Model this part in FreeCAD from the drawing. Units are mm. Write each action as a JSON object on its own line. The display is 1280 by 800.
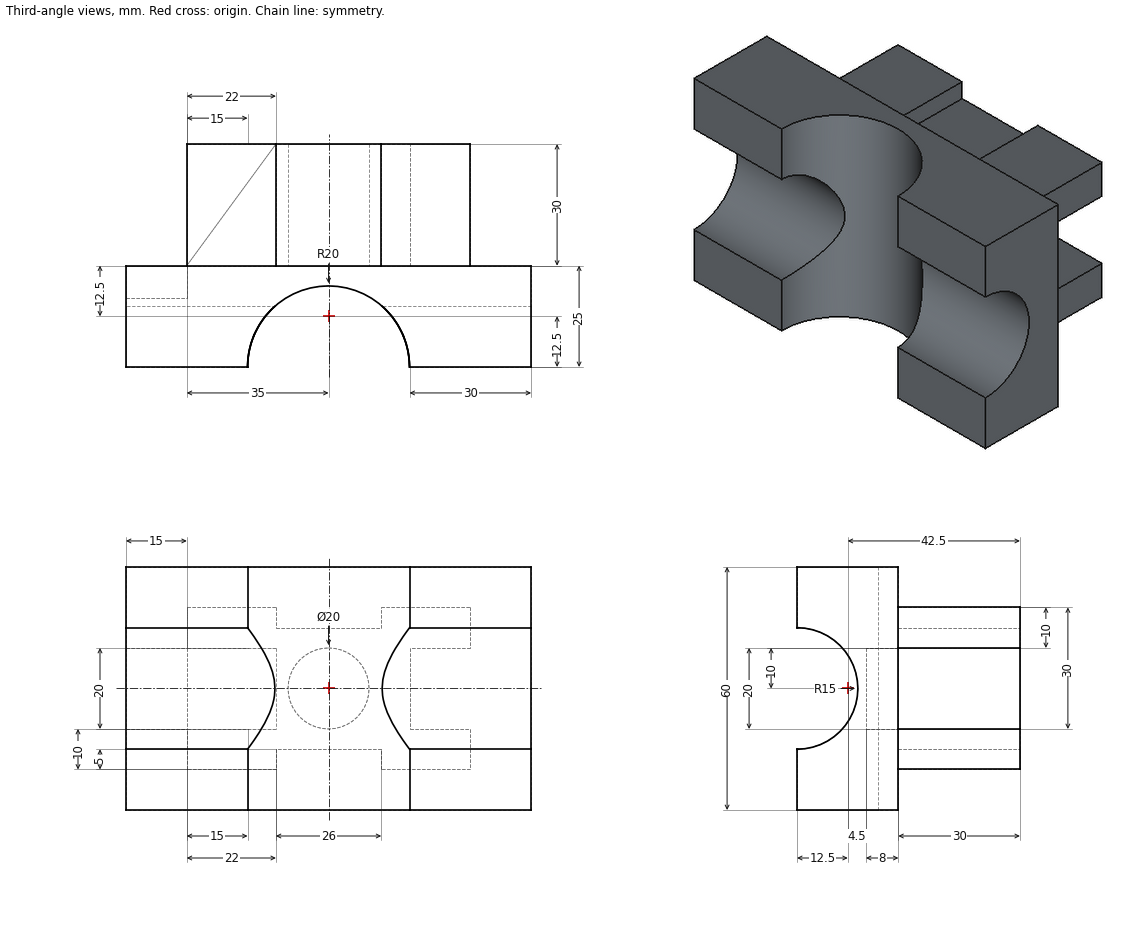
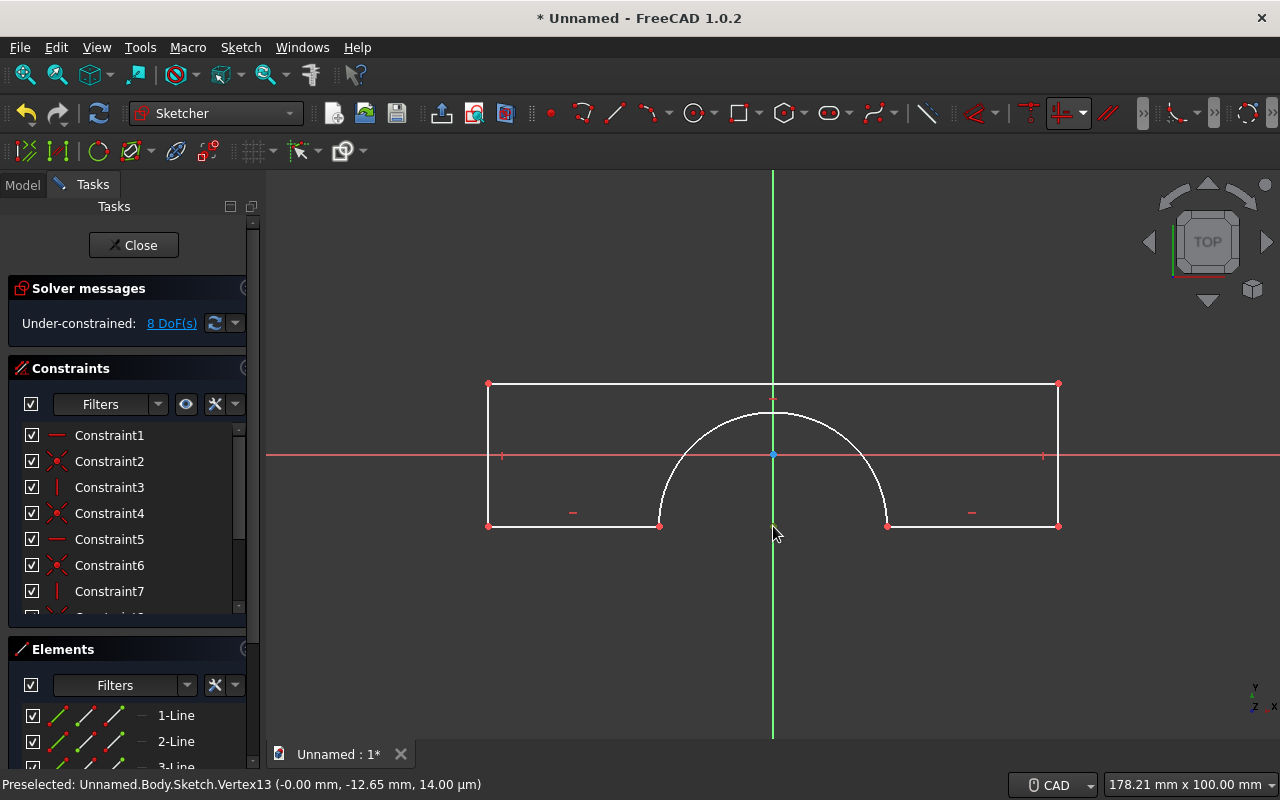
{"action": "left_click", "coordinate": [773, 674]}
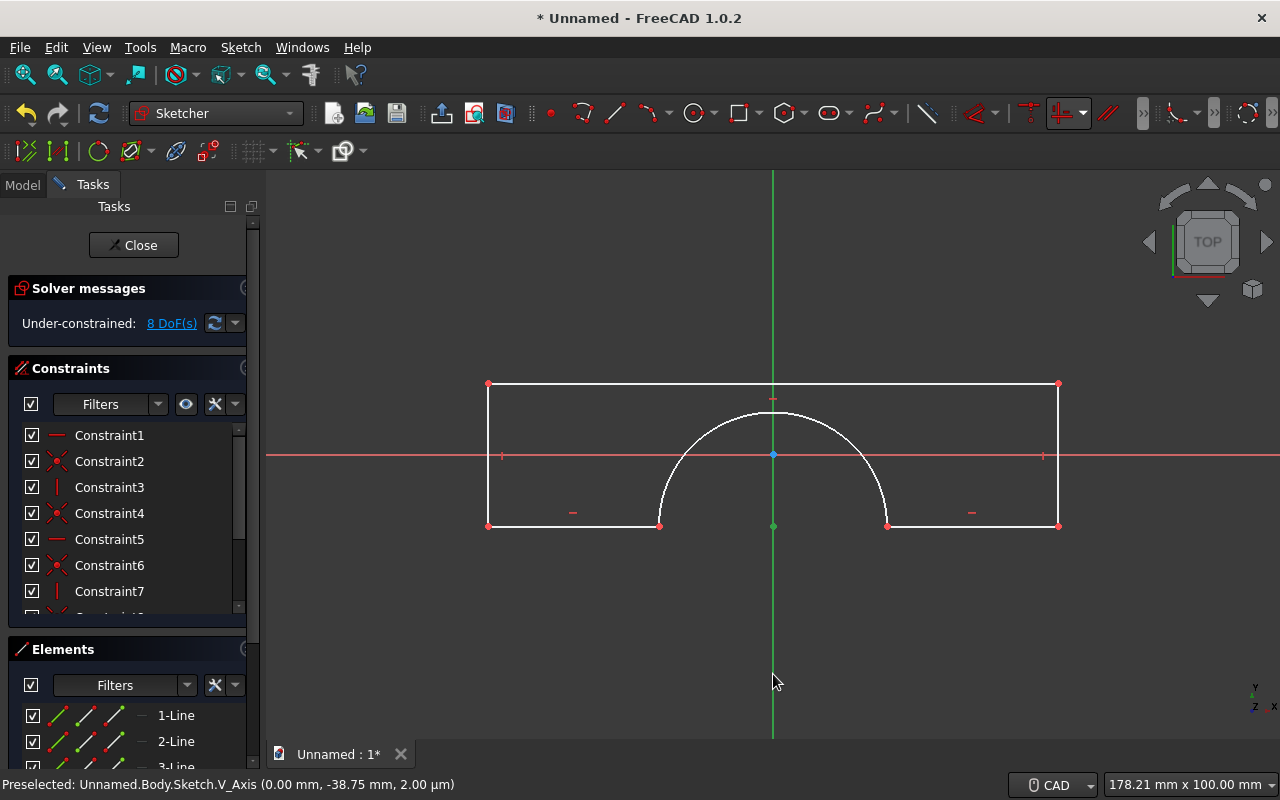
{"action": "key", "text": "c"}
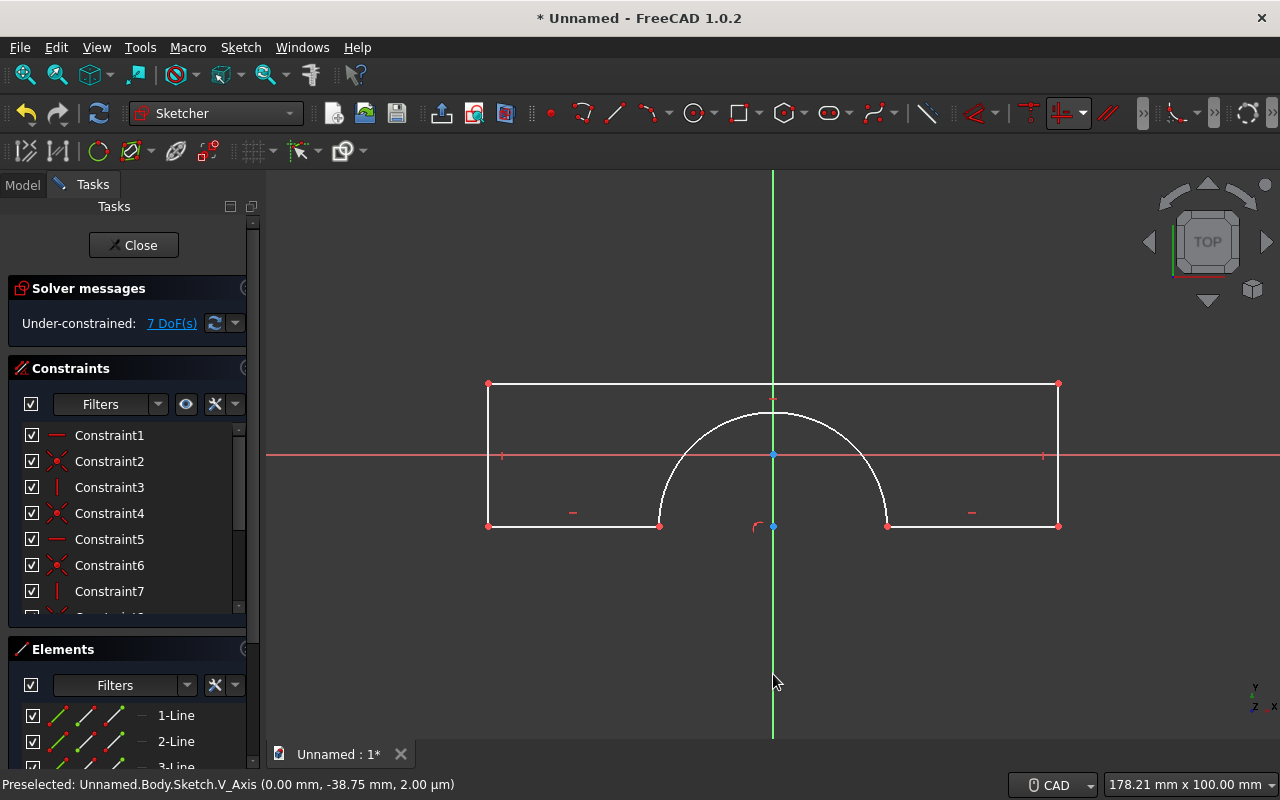
{"action": "left_click", "coordinate": [1058, 527]}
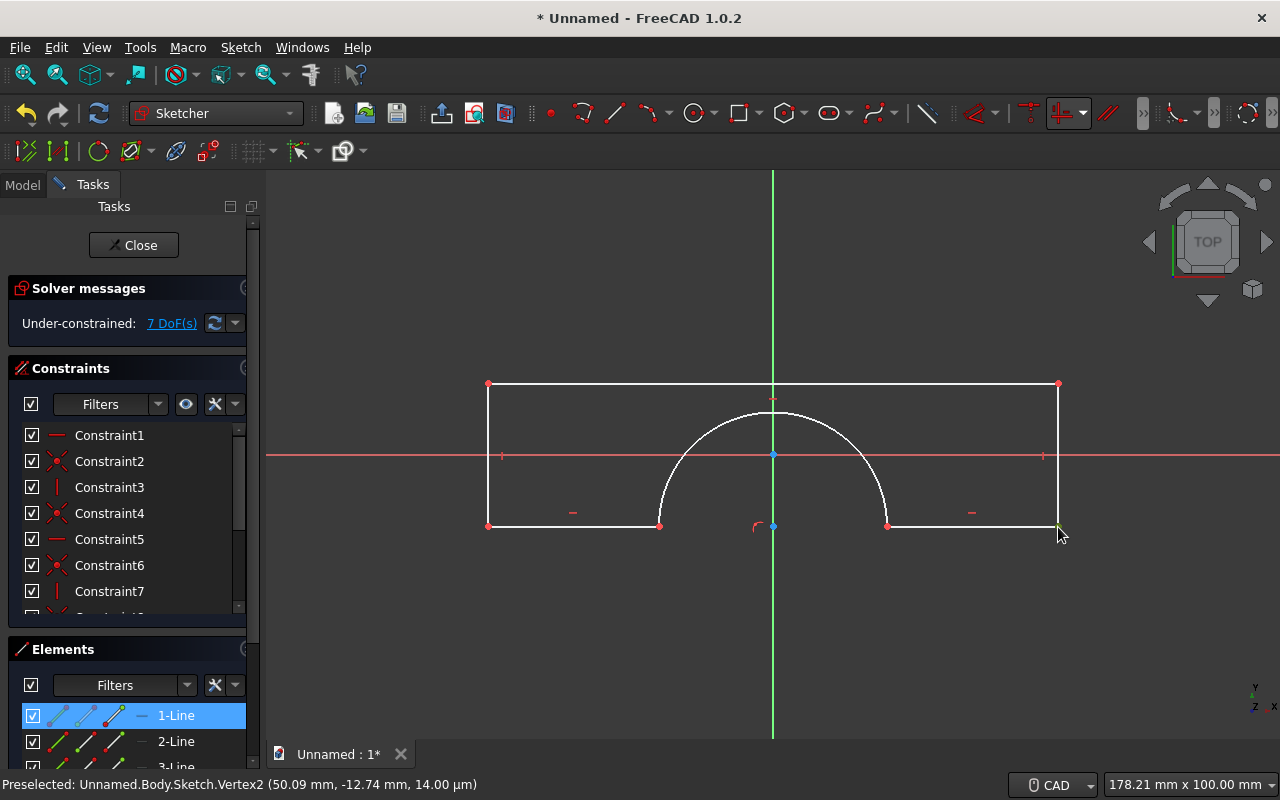
{"action": "left_click", "coordinate": [488, 527]}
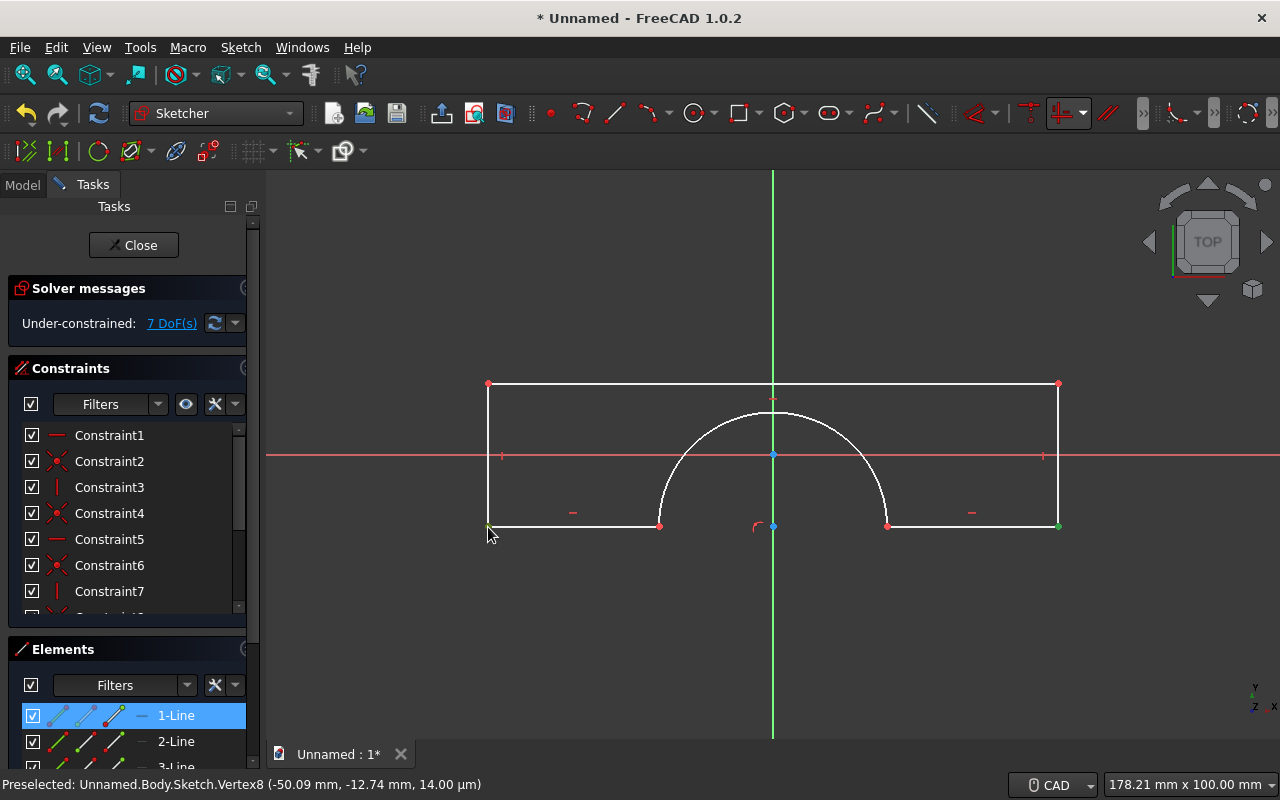
{"action": "left_click", "coordinate": [773, 674]}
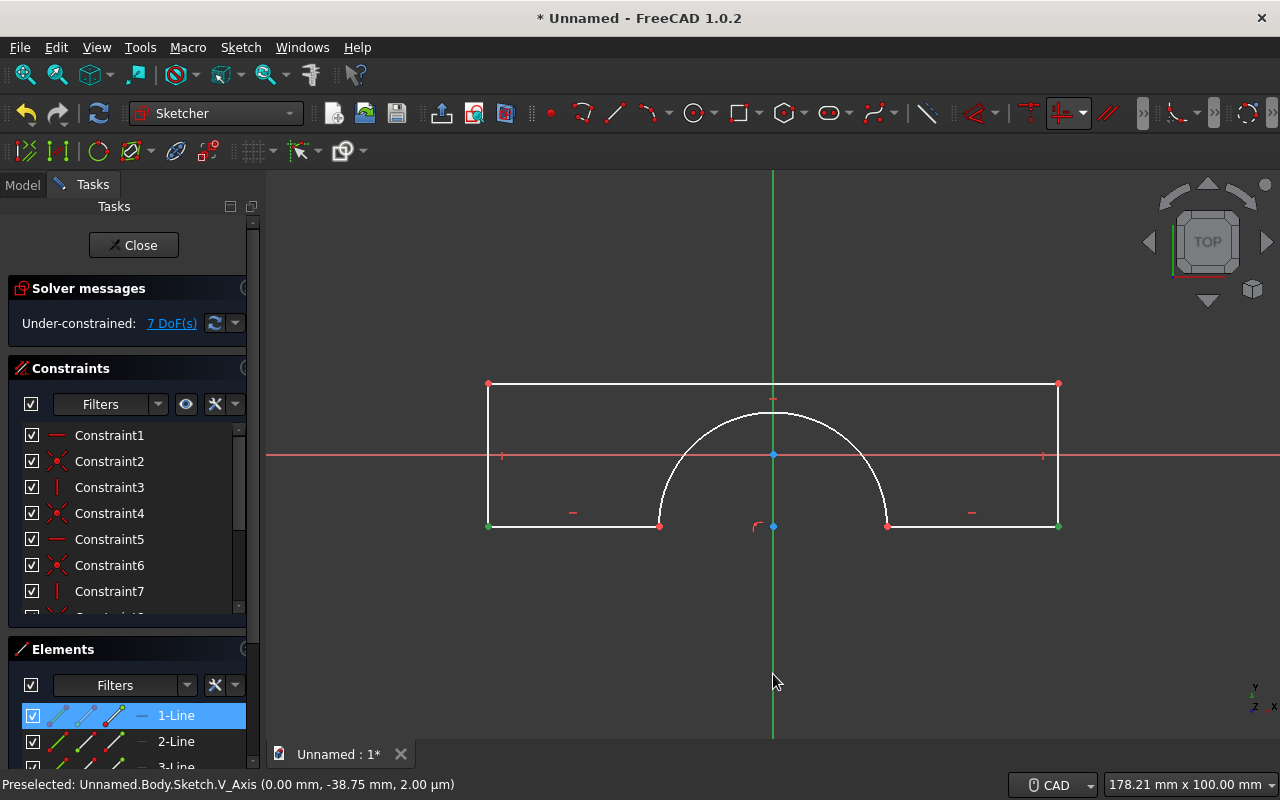
{"action": "key", "text": "s"}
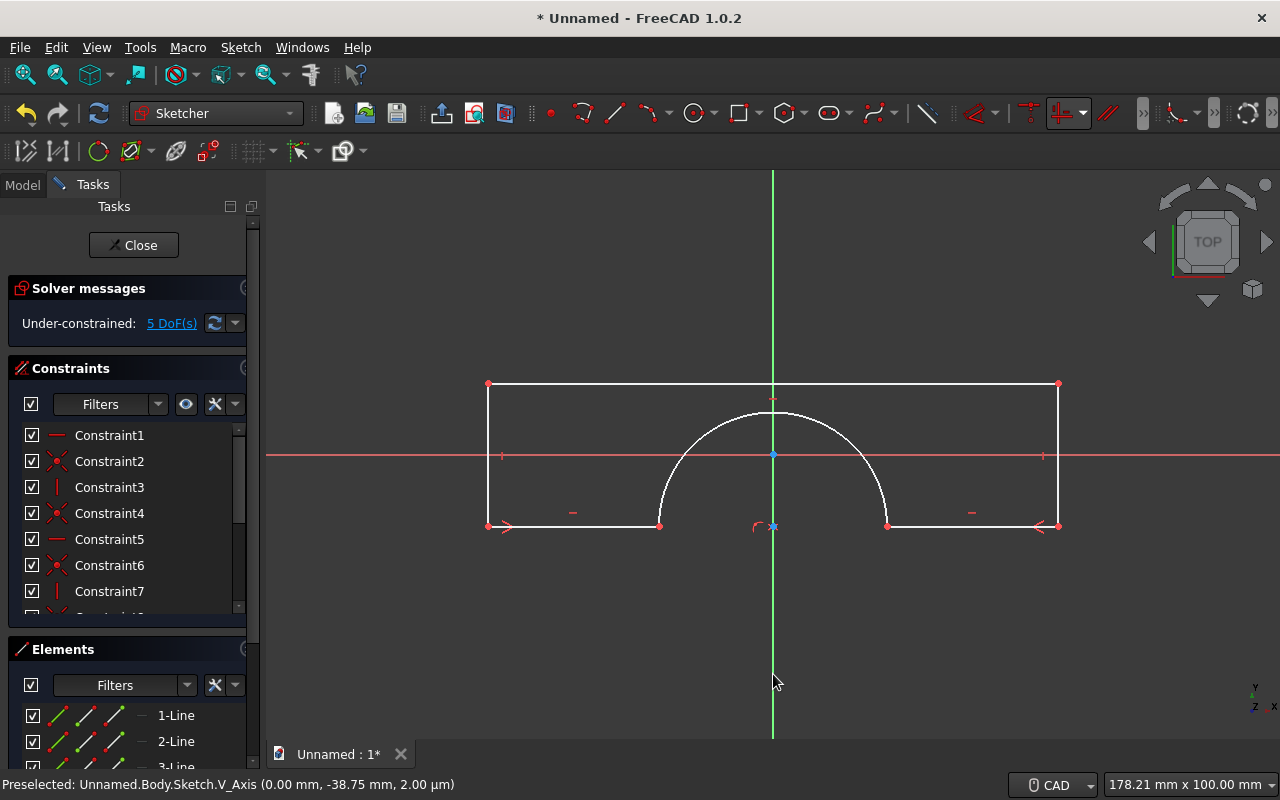
{"action": "left_click", "coordinate": [974, 114]}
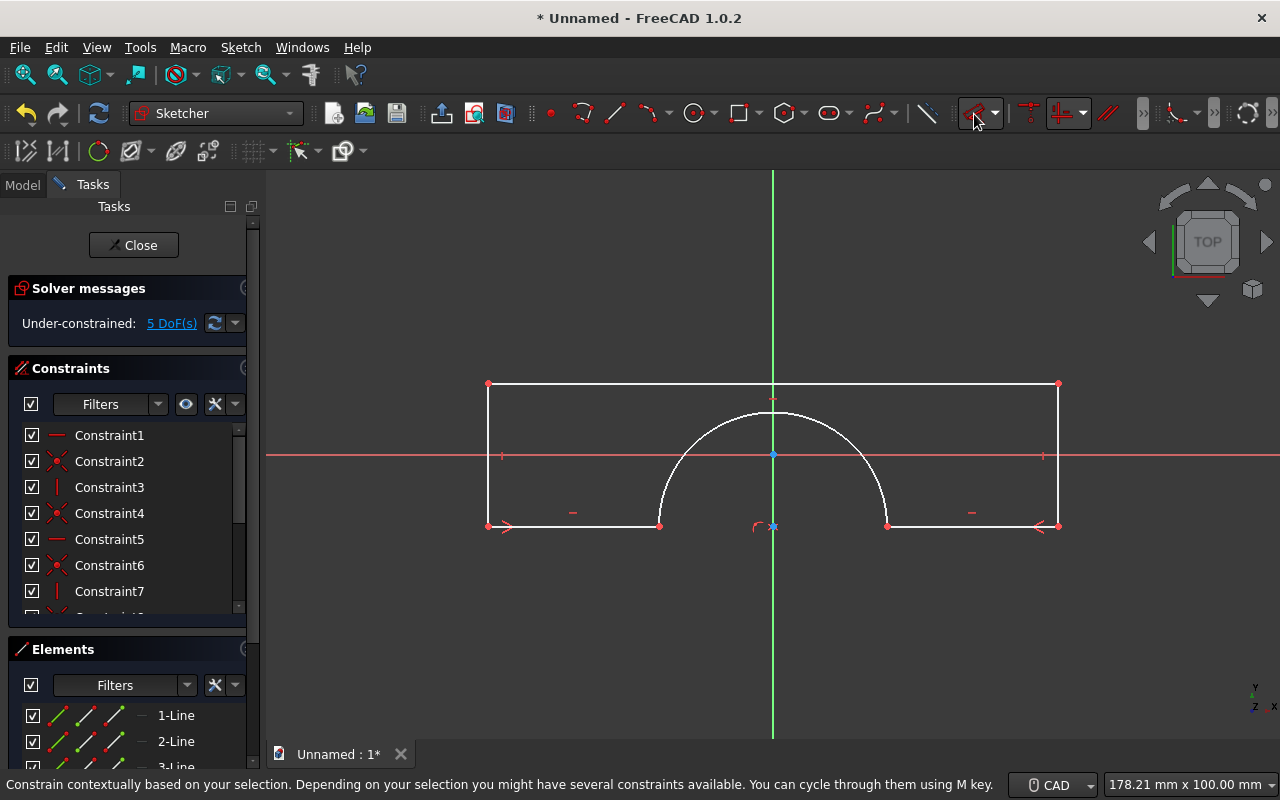
{"action": "left_click", "coordinate": [840, 434]}
{"action": "left_click", "coordinate": [859, 408]}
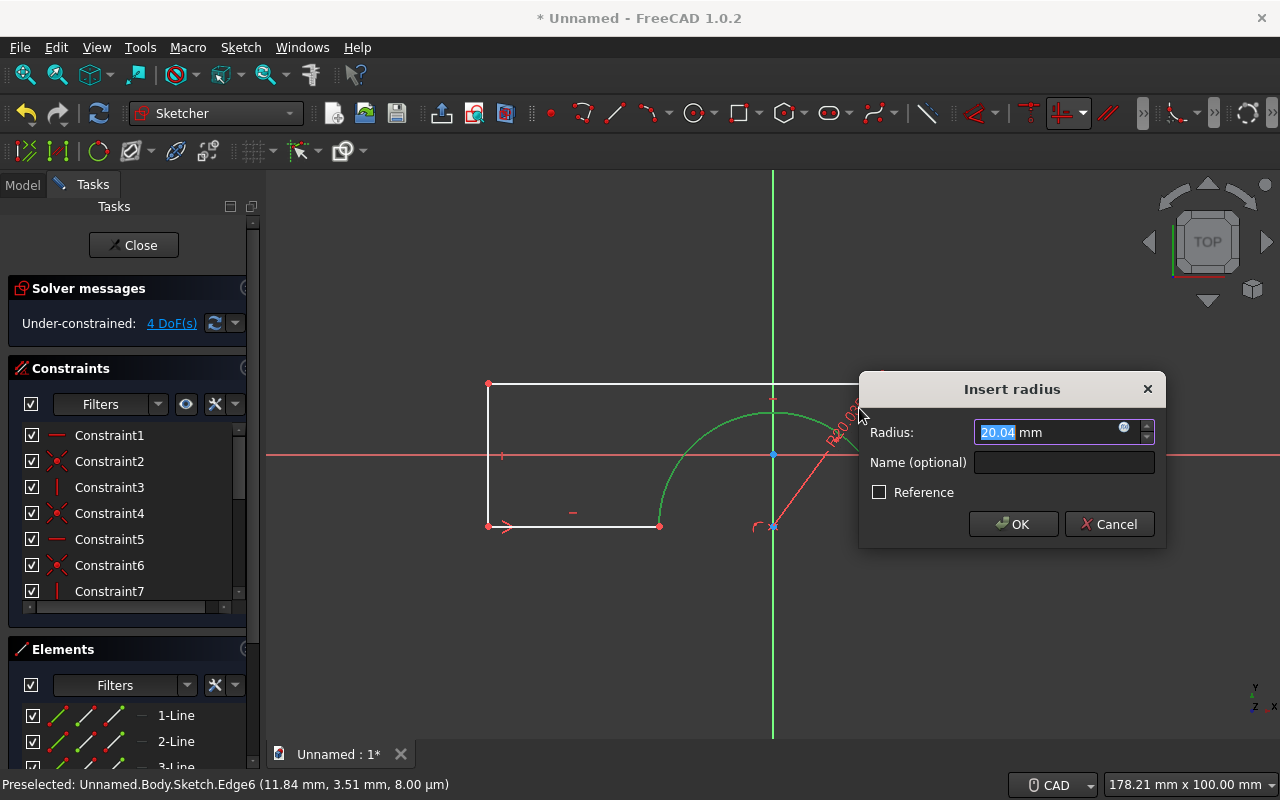
{"action": "type", "text": "20"}
{"action": "key", "text": "Return"}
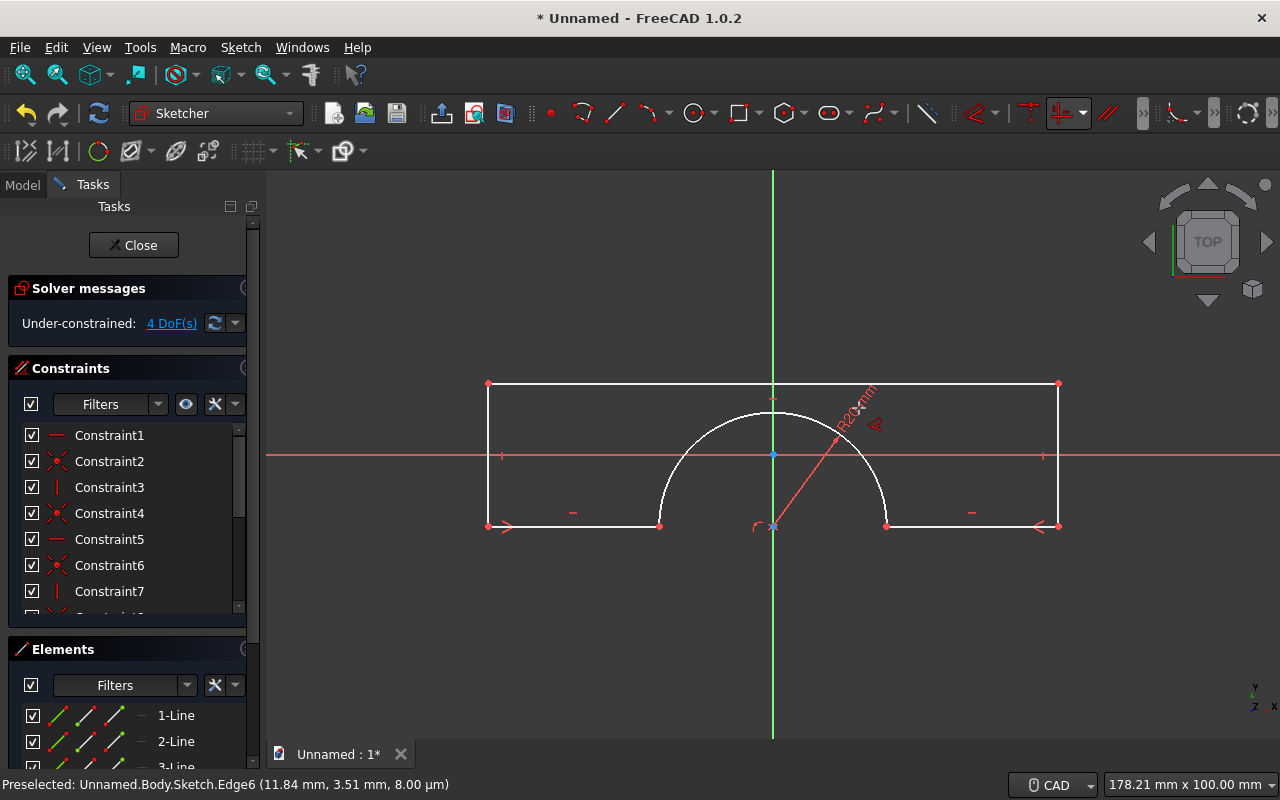
{"action": "left_click", "coordinate": [938, 527]}
{"action": "left_click", "coordinate": [972, 561]}